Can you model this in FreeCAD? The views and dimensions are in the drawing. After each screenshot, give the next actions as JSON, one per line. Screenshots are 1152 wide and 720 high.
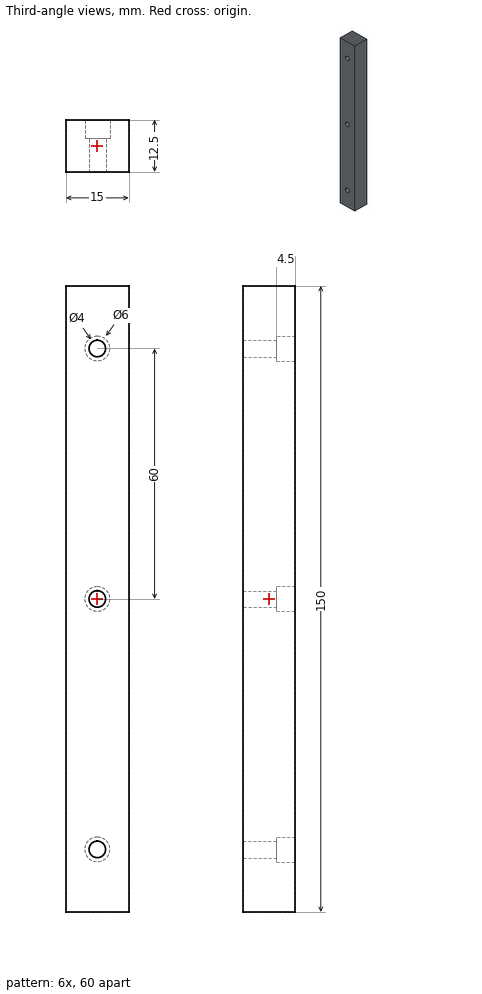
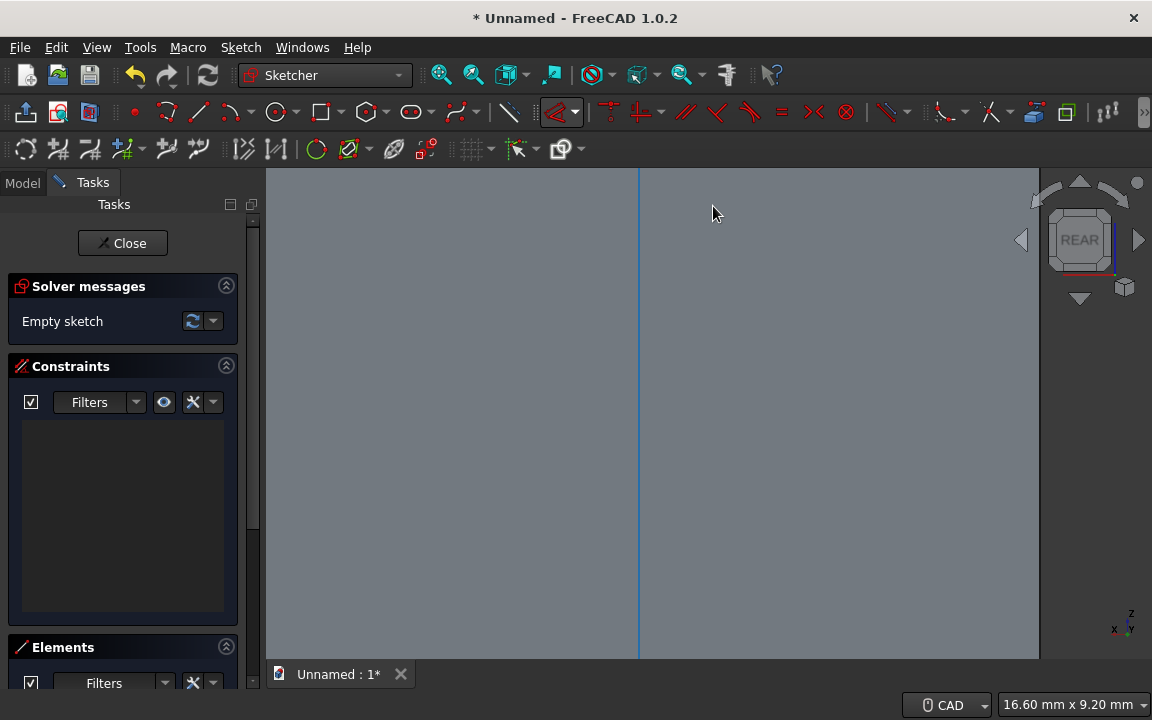
{"action": "left_click", "coordinate": [276, 112]}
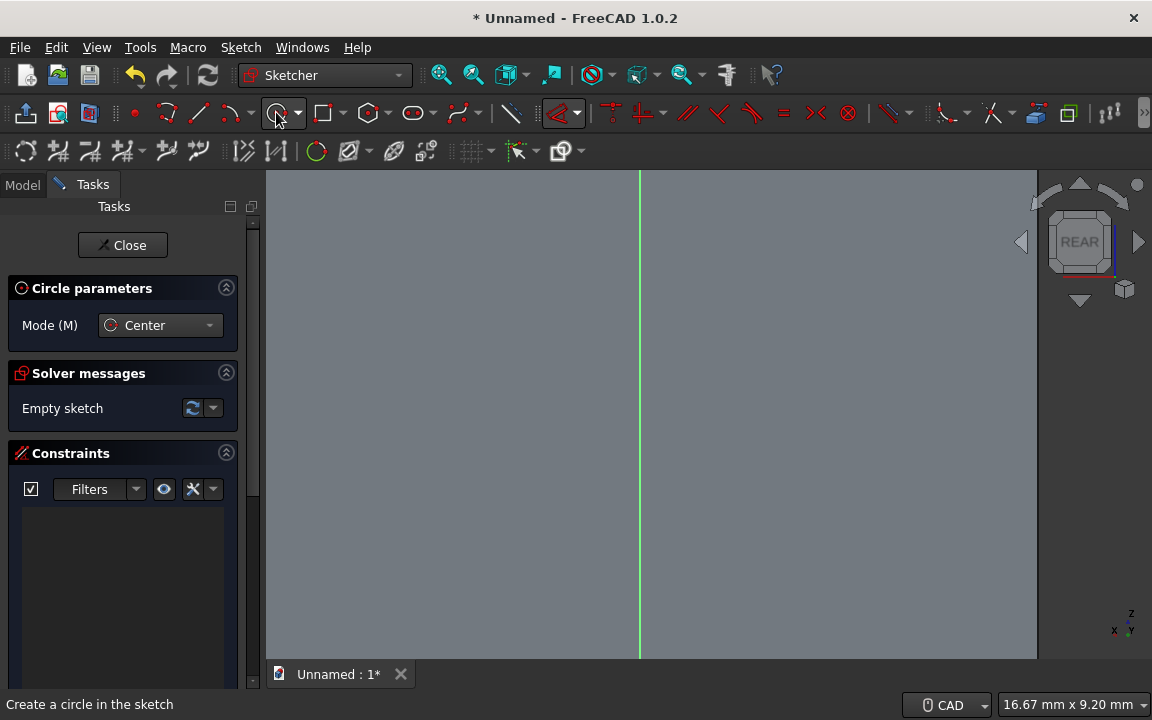
{"action": "left_click", "coordinate": [640, 415]}
{"action": "left_click", "coordinate": [752, 303]}
{"action": "key", "text": "Escape"}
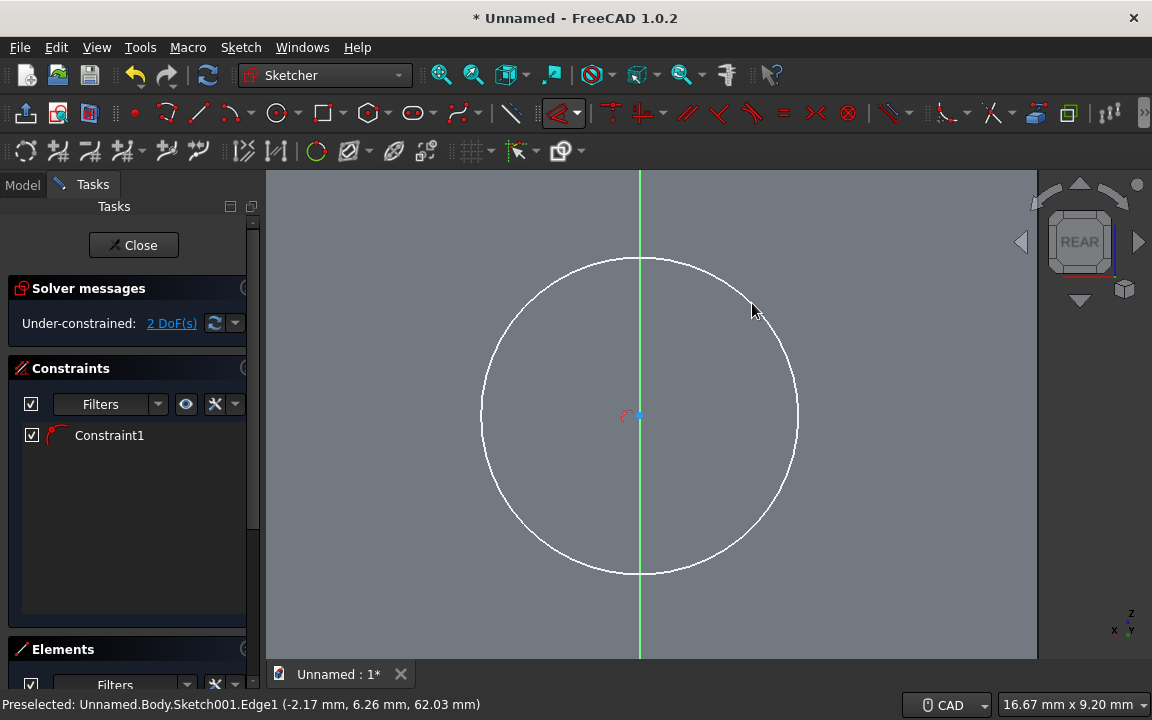
{"action": "left_click", "coordinate": [752, 304]}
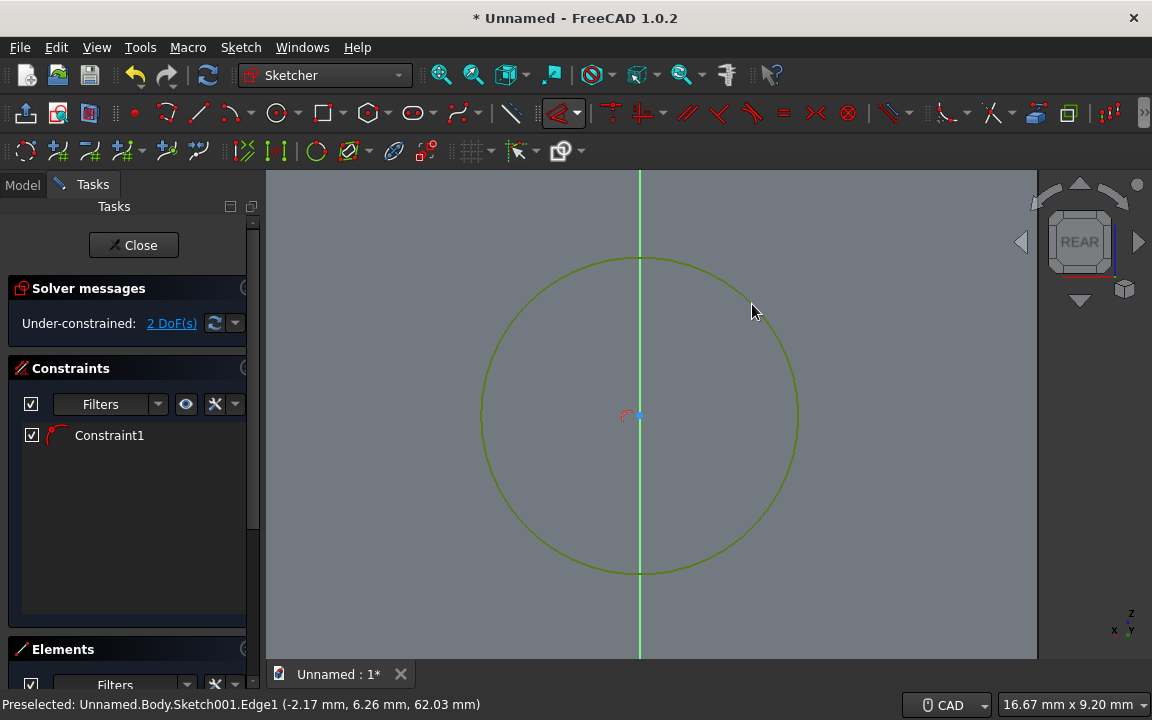
{"action": "key", "text": "k o"}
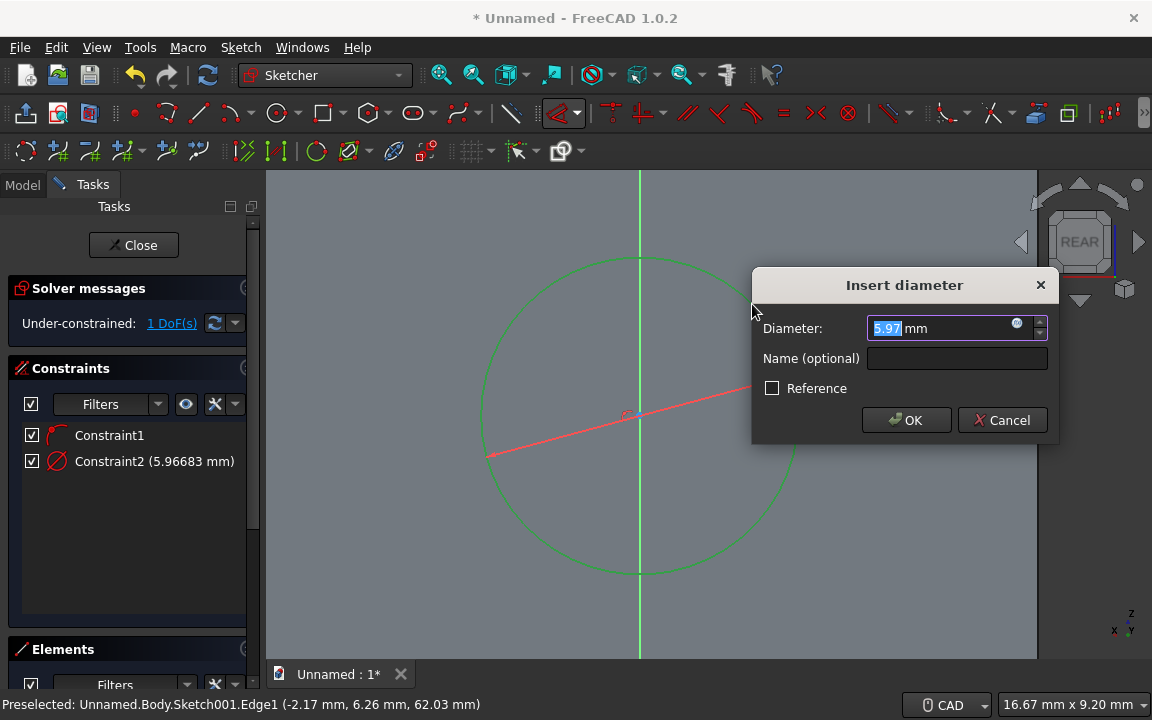
{"action": "type", "text": "6"}
{"action": "key", "text": "Return"}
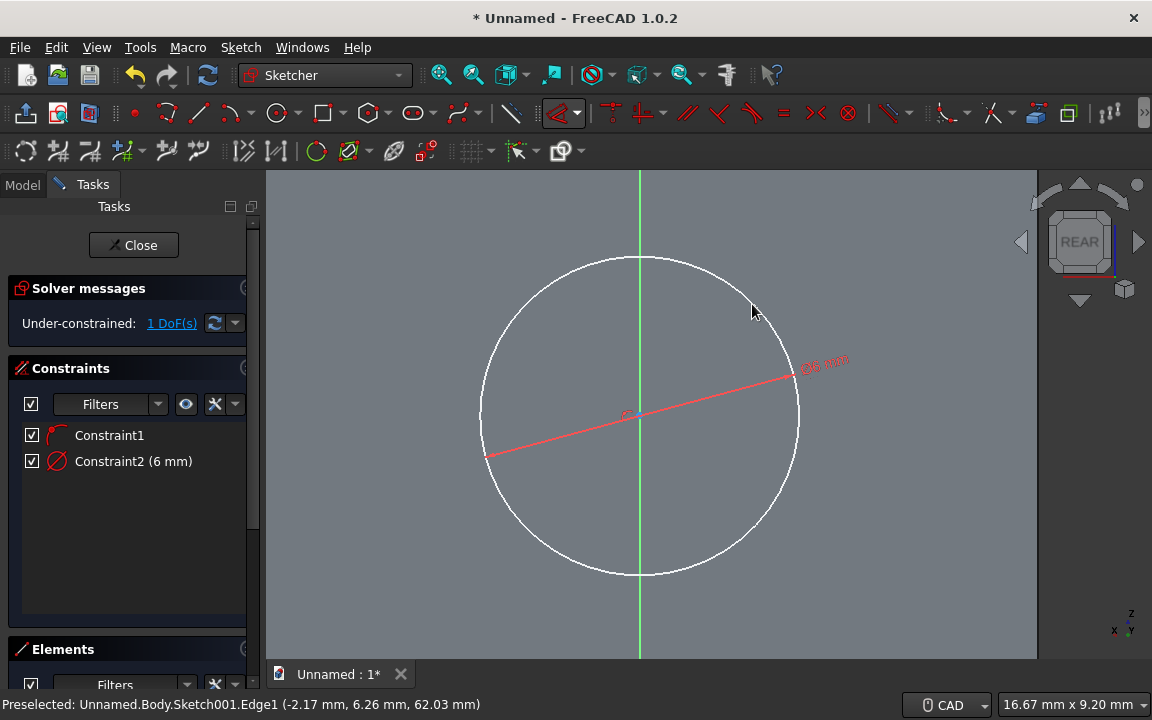
{"action": "left_click", "coordinate": [640, 416]}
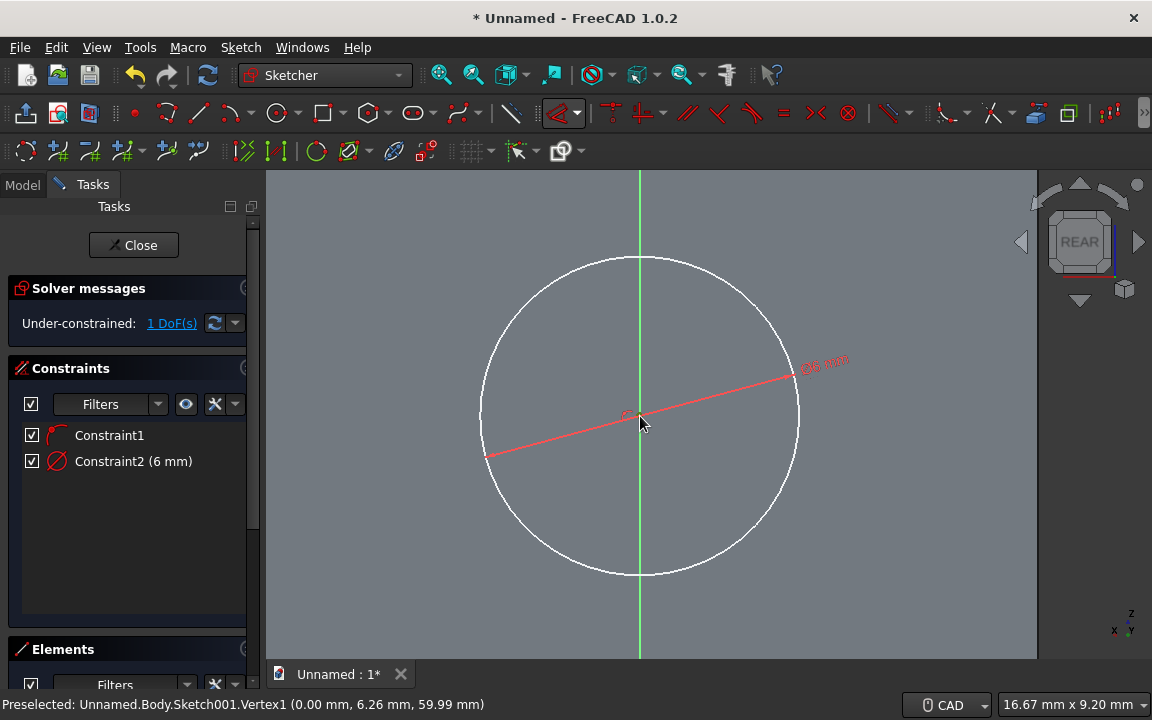
{"action": "key", "text": "i"}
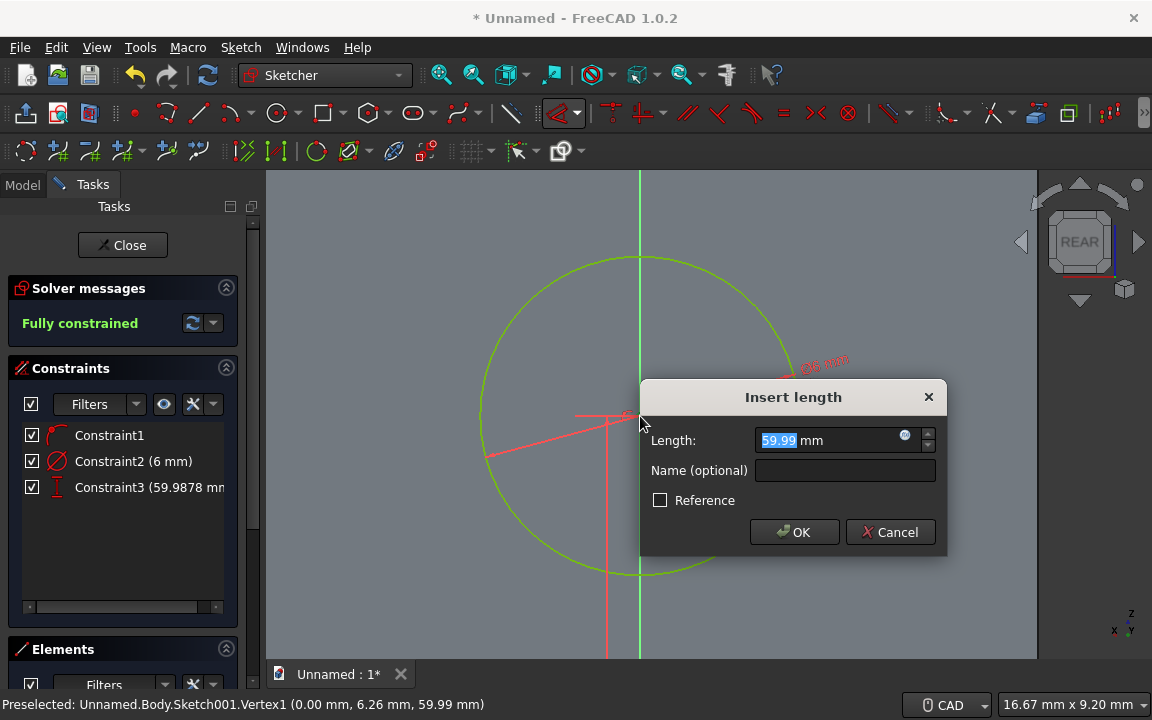
{"action": "type", "text": "60"}
{"action": "key", "text": "Return"}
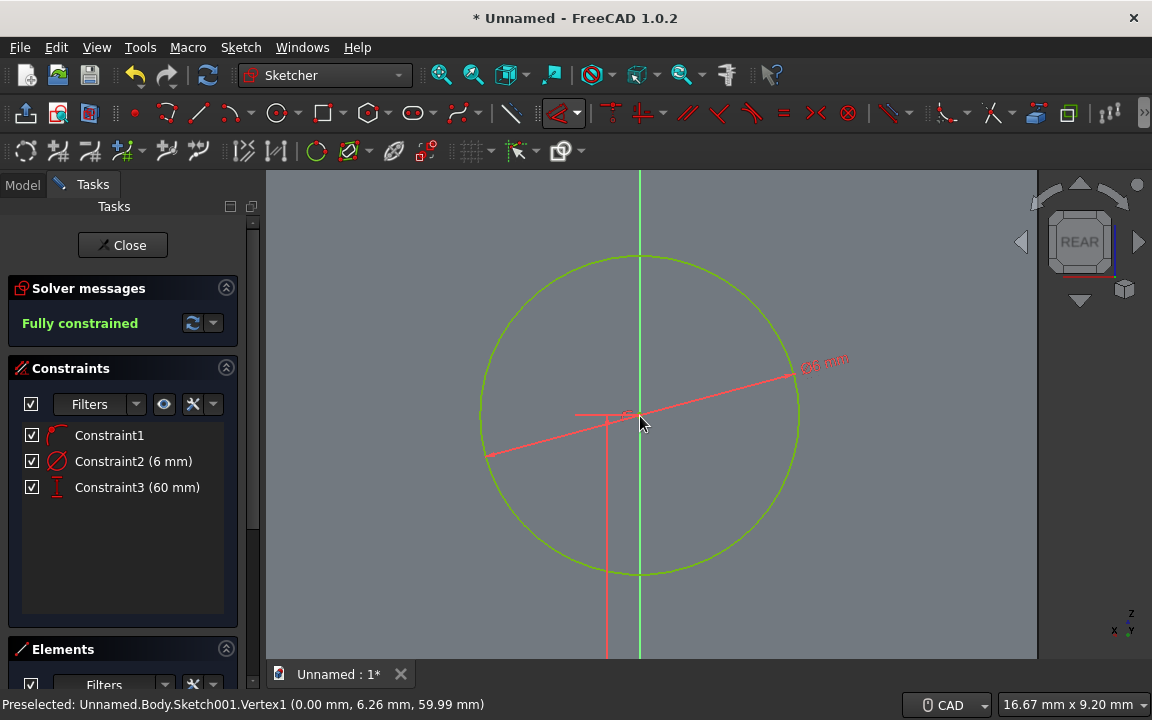
{"action": "left_click", "coordinate": [123, 245]}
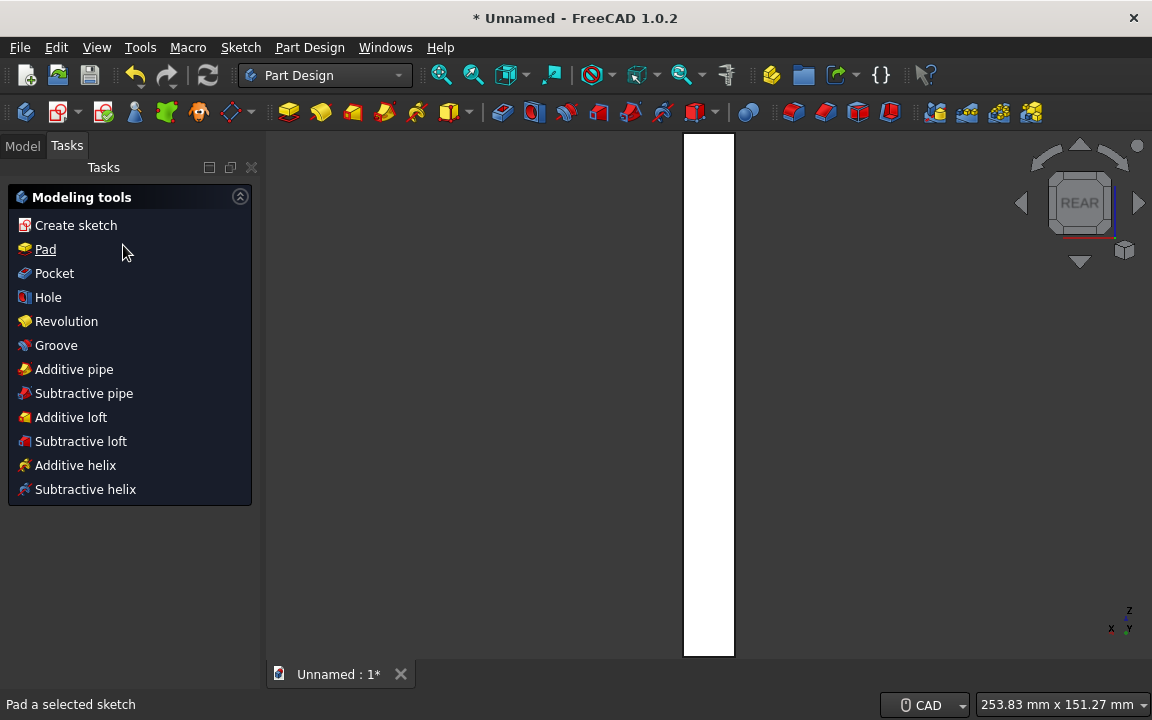
{"action": "left_click", "coordinate": [504, 112]}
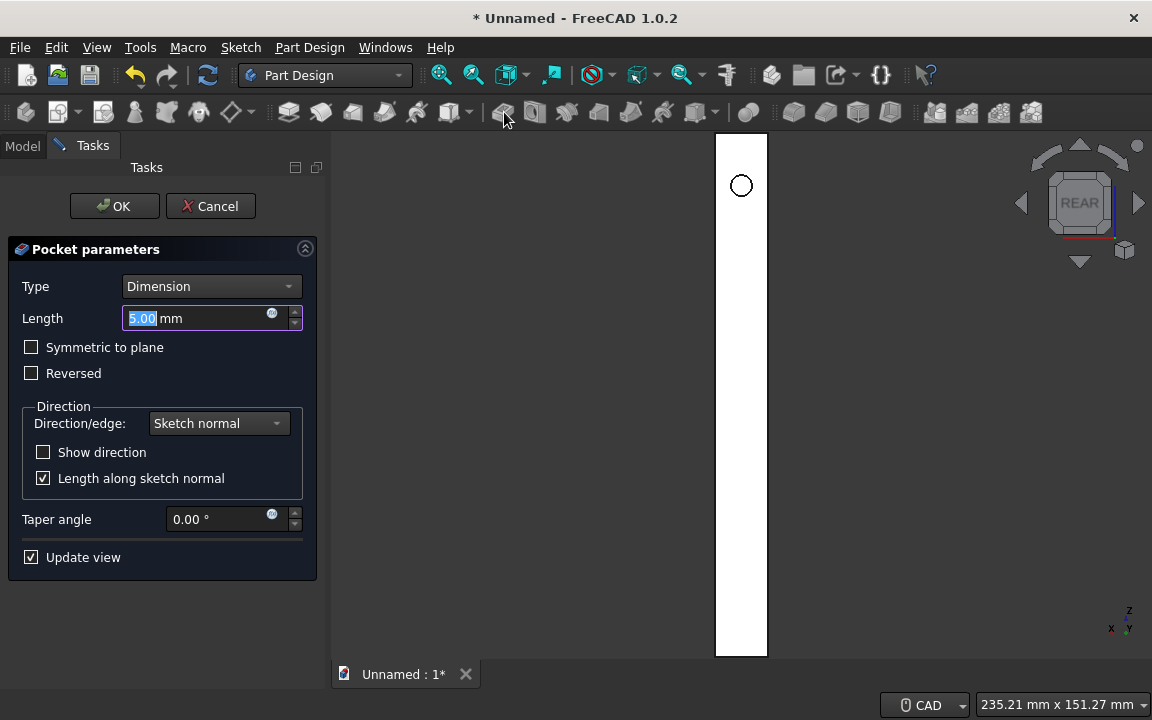
{"action": "type", "text": "4.5"}
{"action": "key", "text": "Tab"}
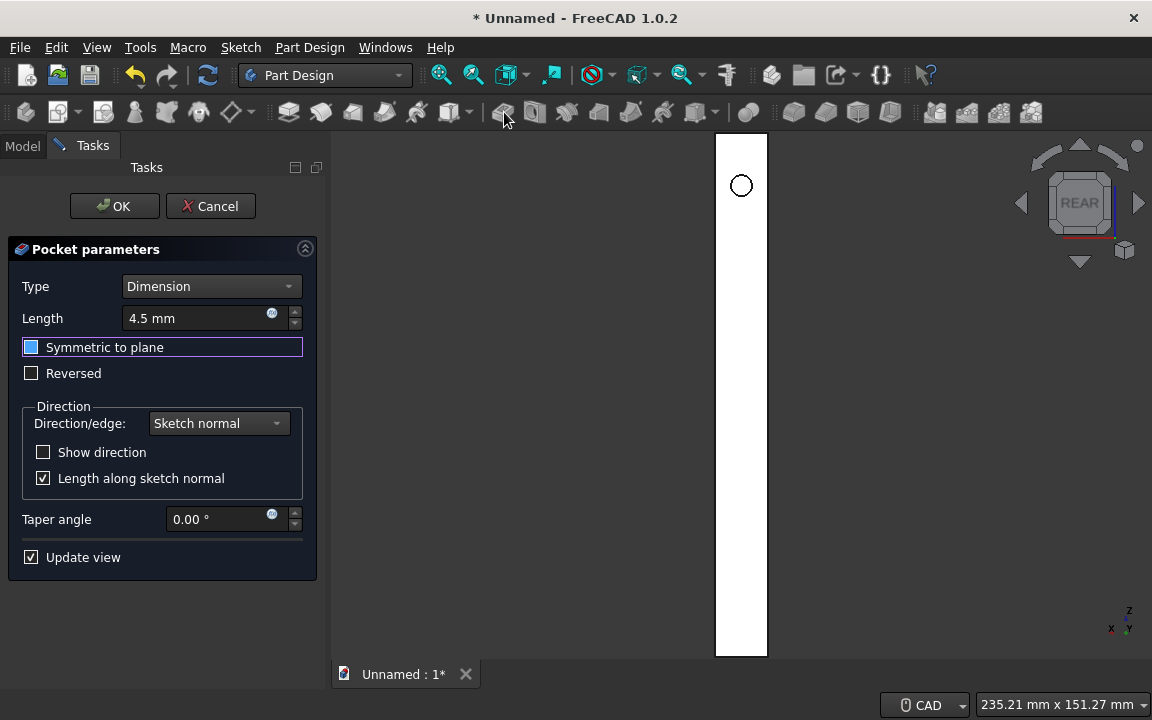
{"action": "left_click", "coordinate": [115, 206]}